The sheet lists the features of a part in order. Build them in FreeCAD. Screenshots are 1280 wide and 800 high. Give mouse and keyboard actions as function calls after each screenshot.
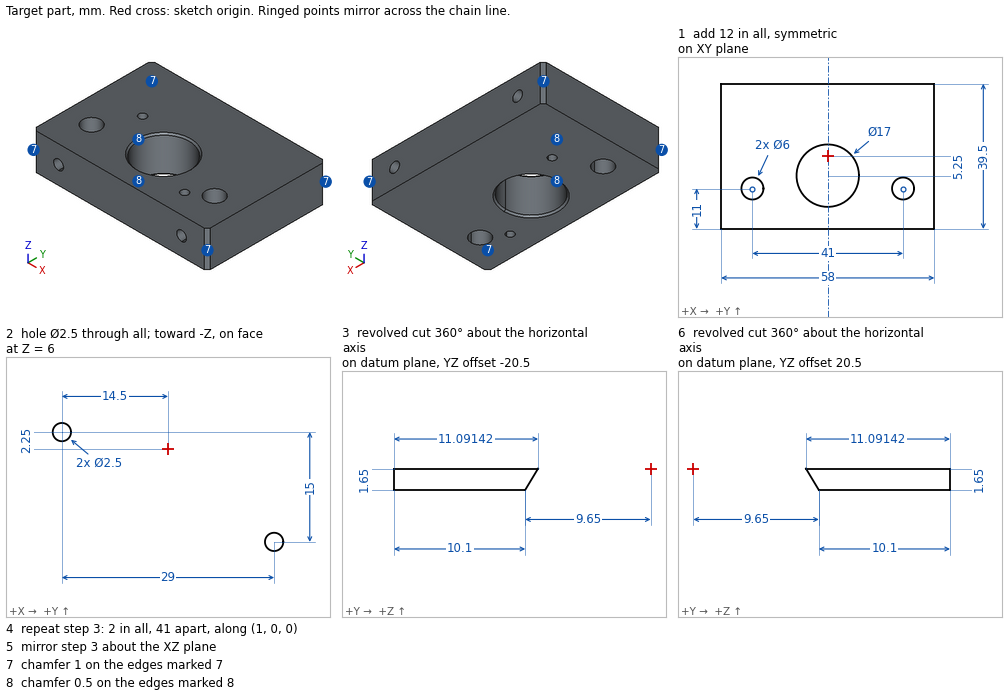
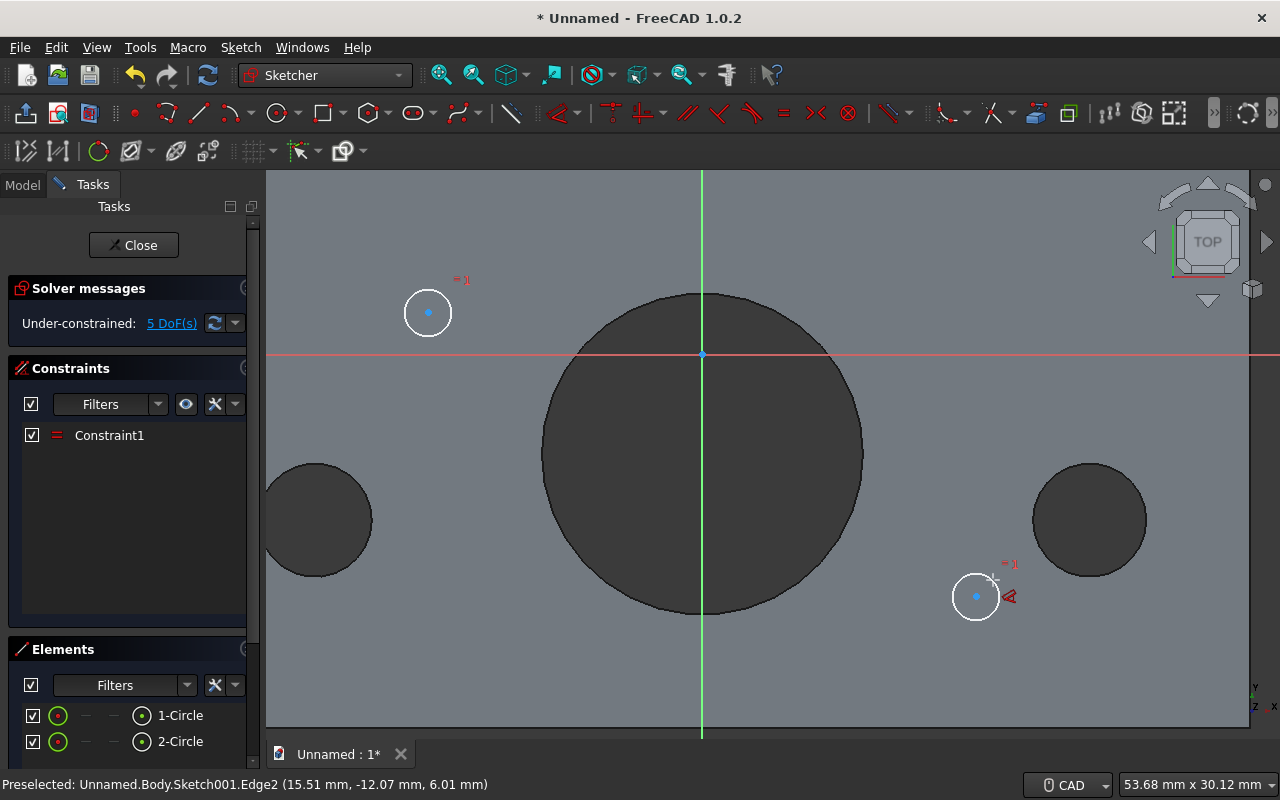
click(444, 296)
click(466, 273)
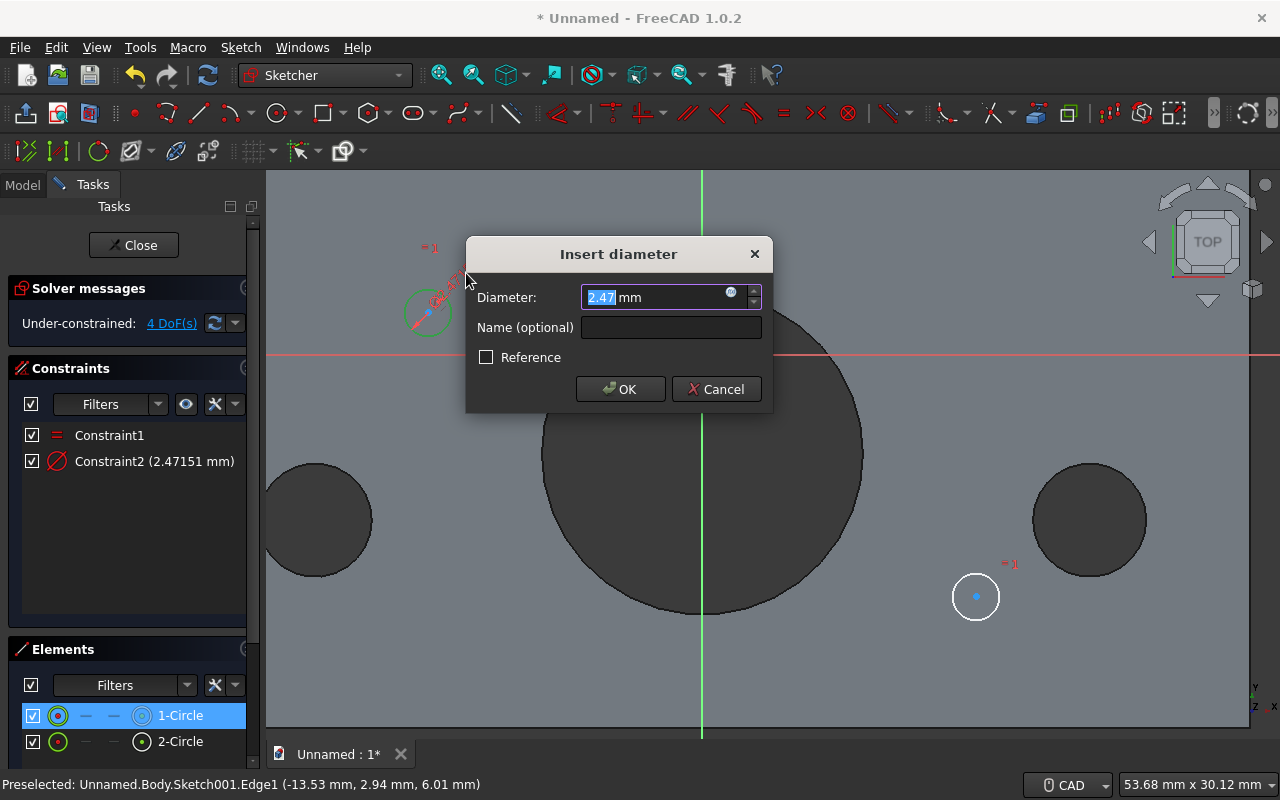
text(2.5)
key(Return)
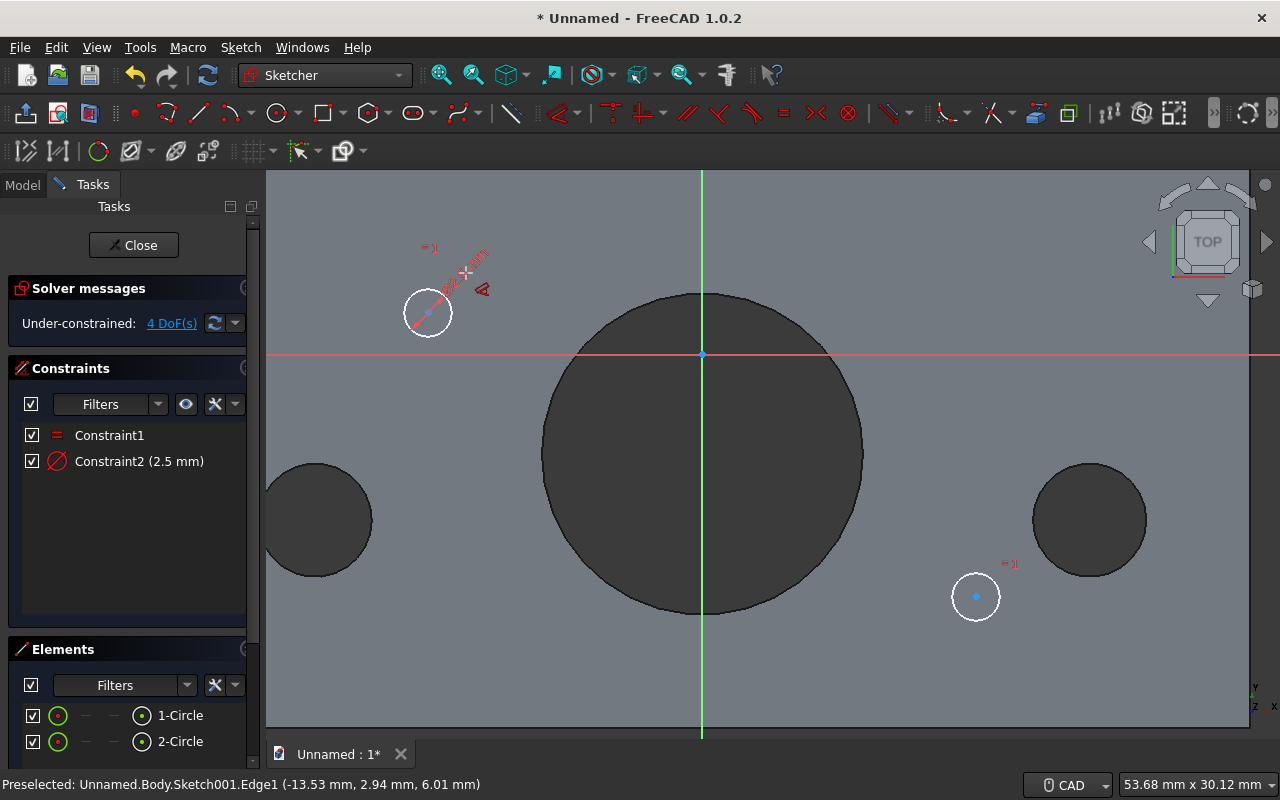
click(428, 313)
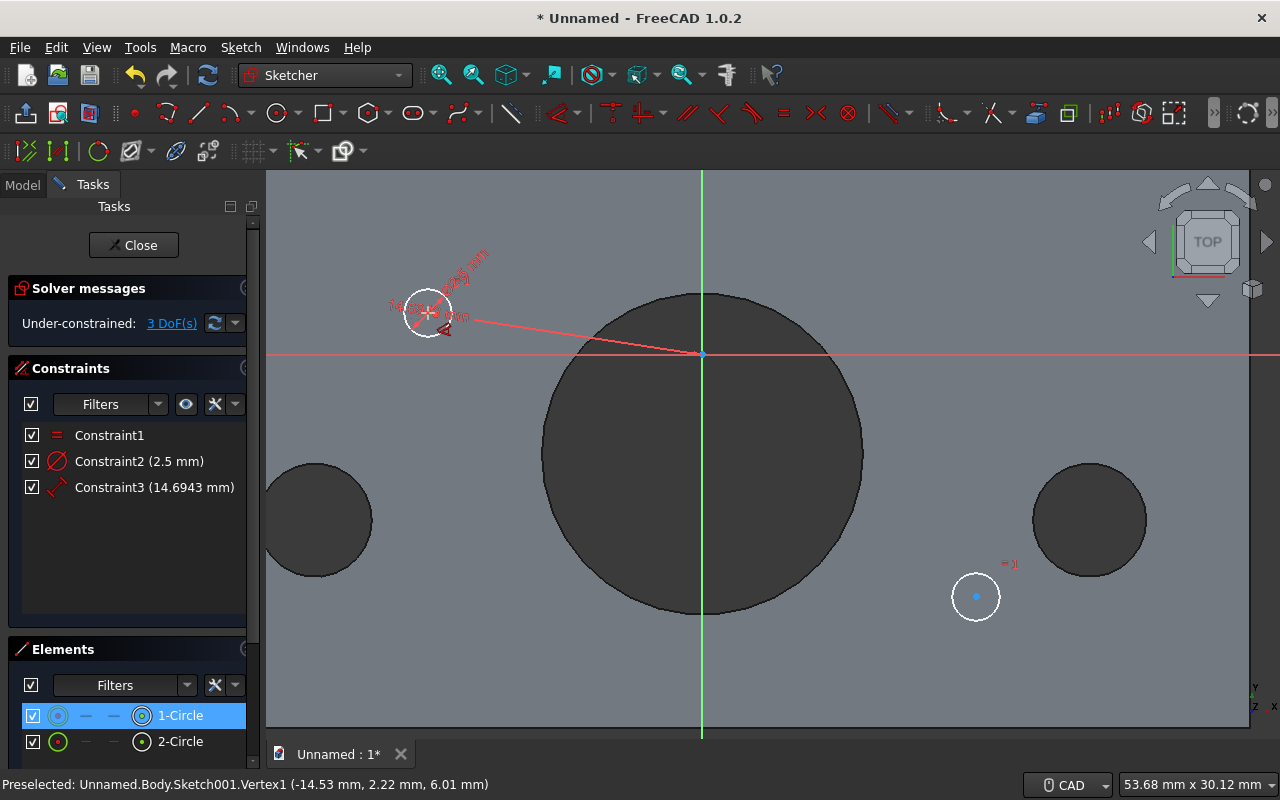
click(976, 597)
click(576, 631)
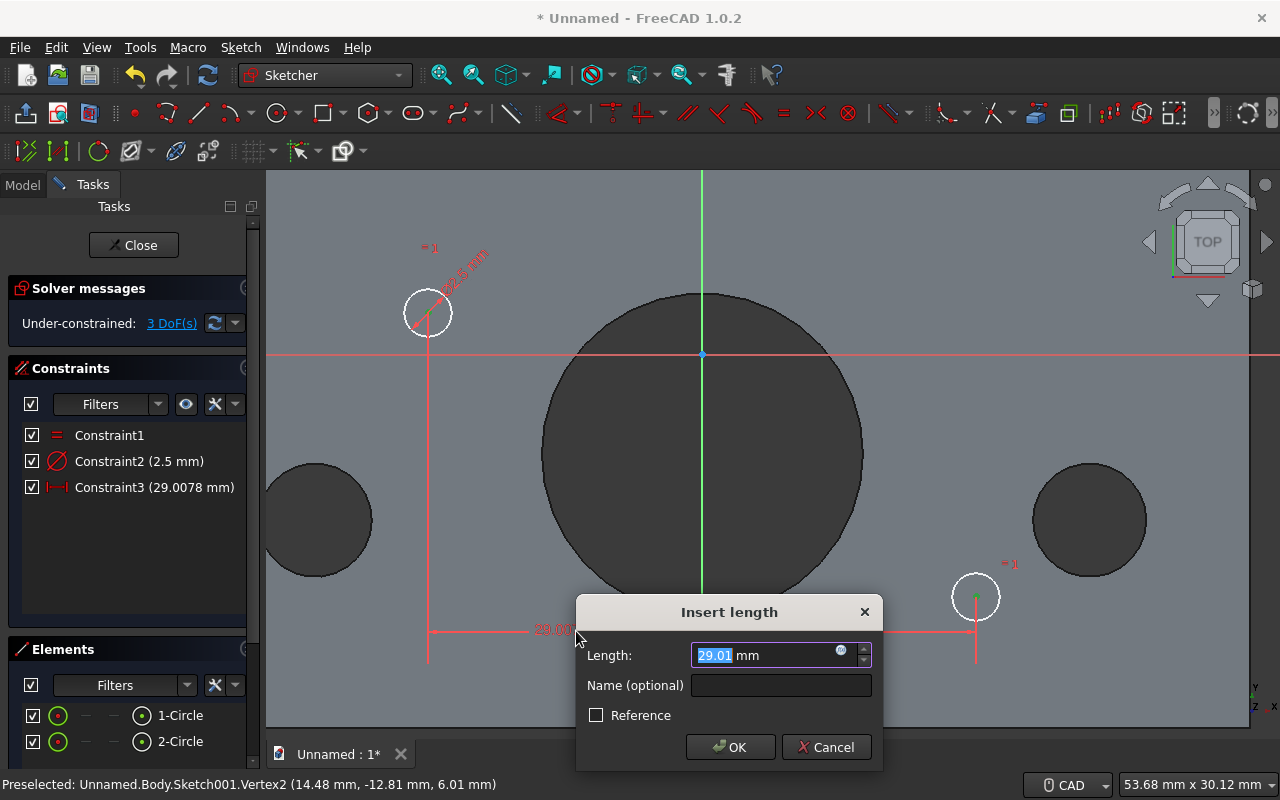
text(29)
key(Return)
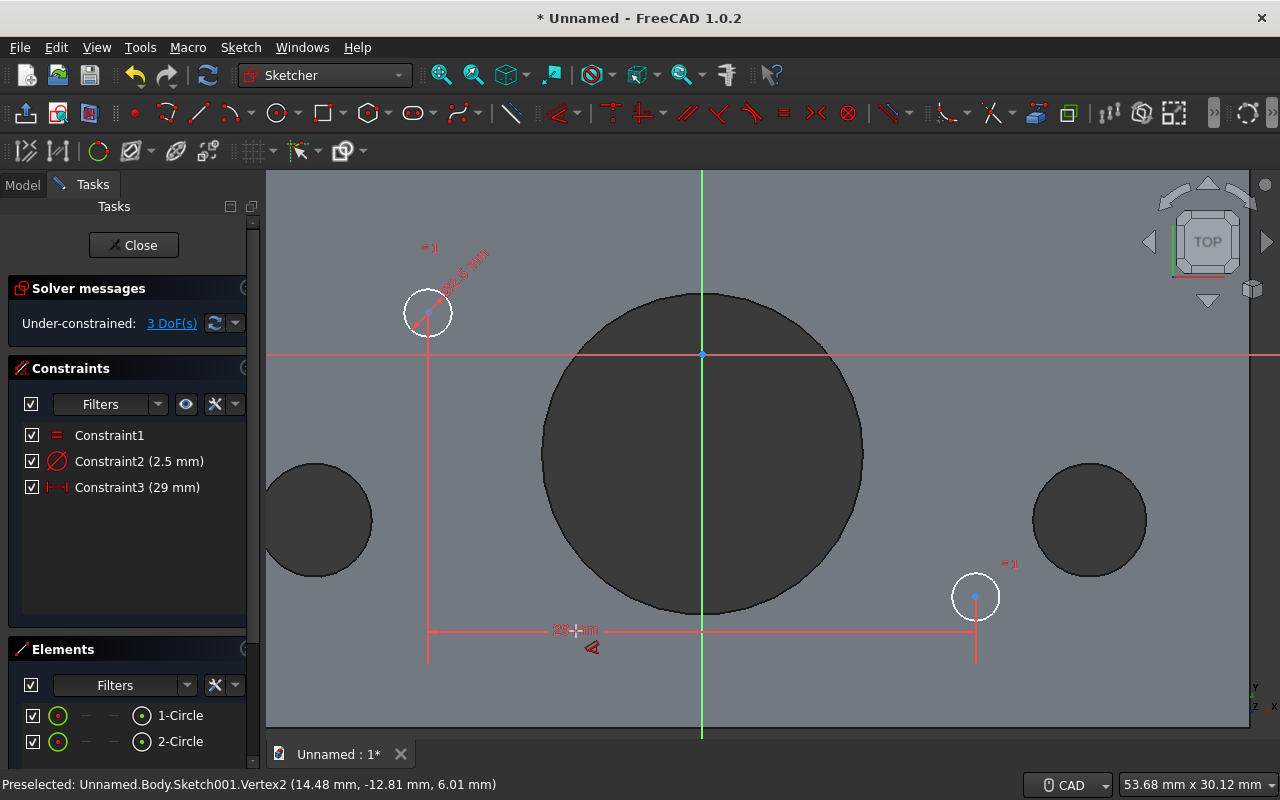
click(428, 313)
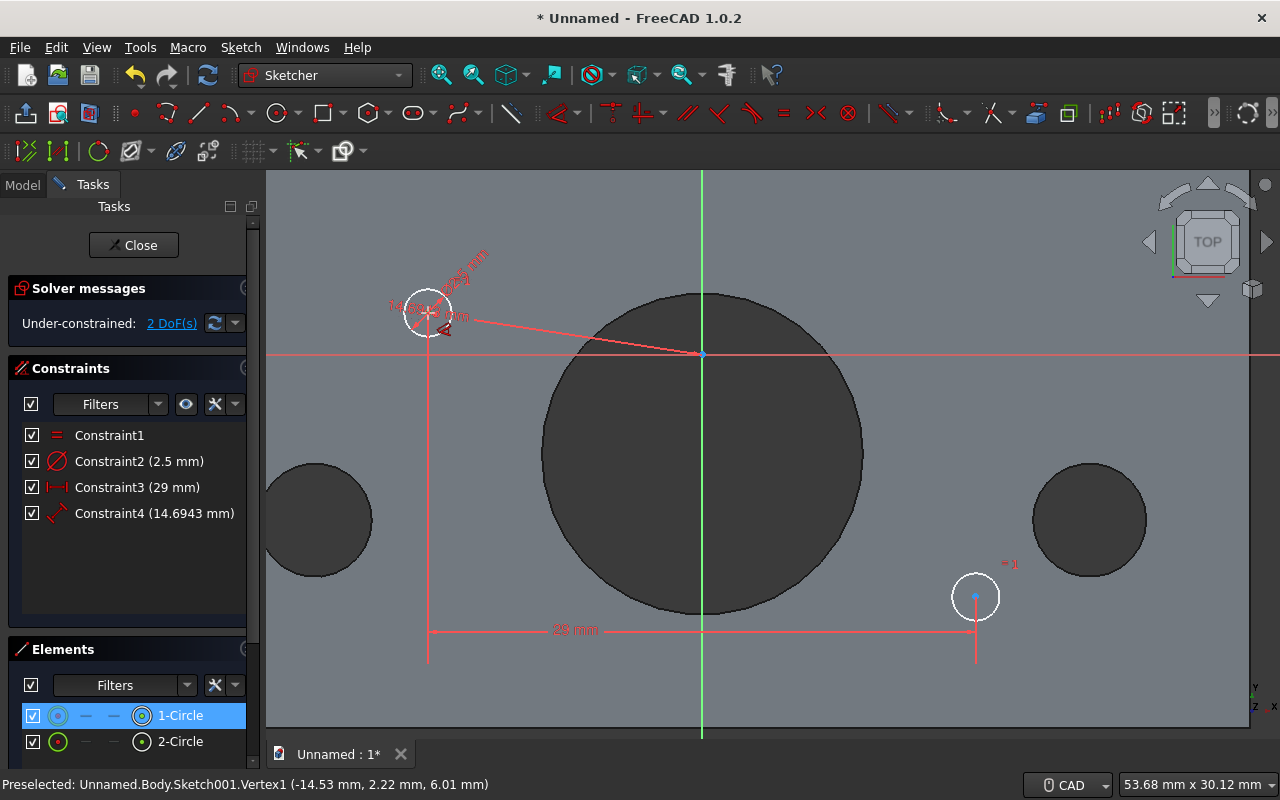
click(976, 597)
click(394, 455)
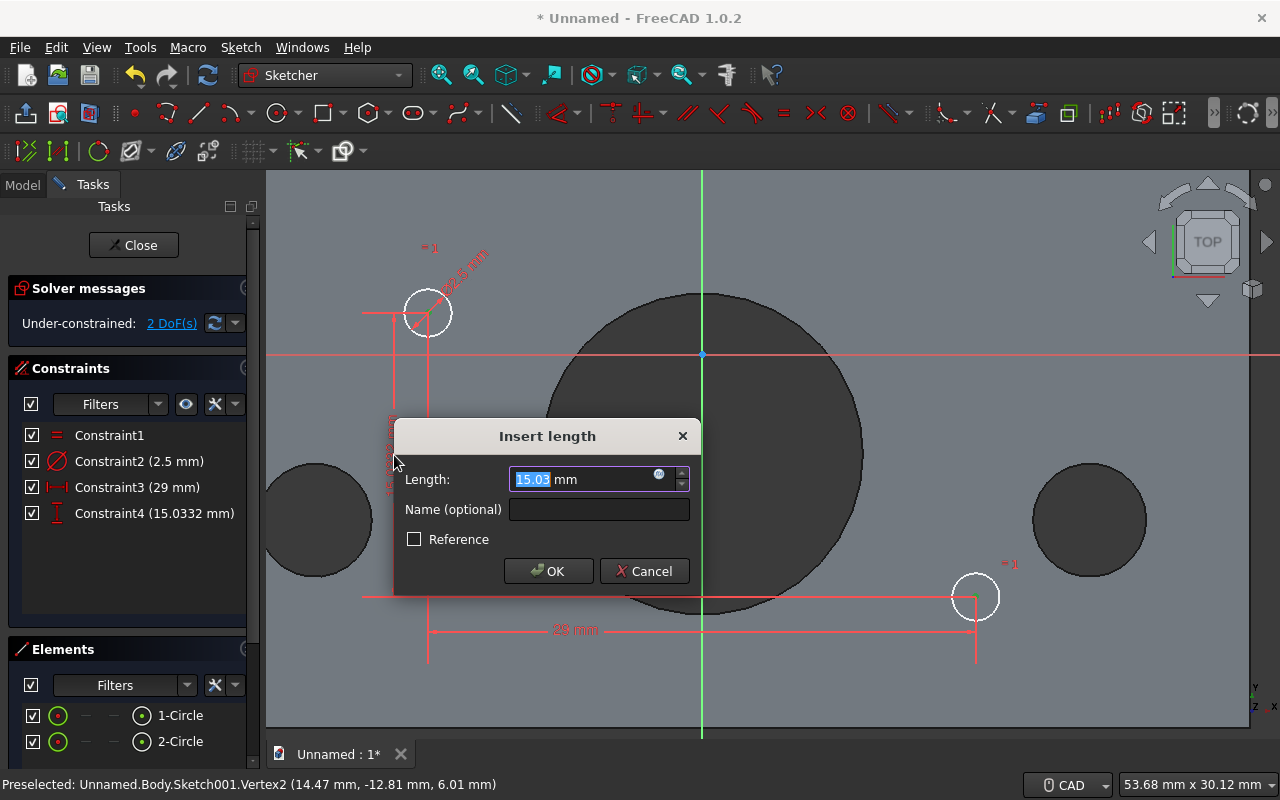
text(15)
key(Return)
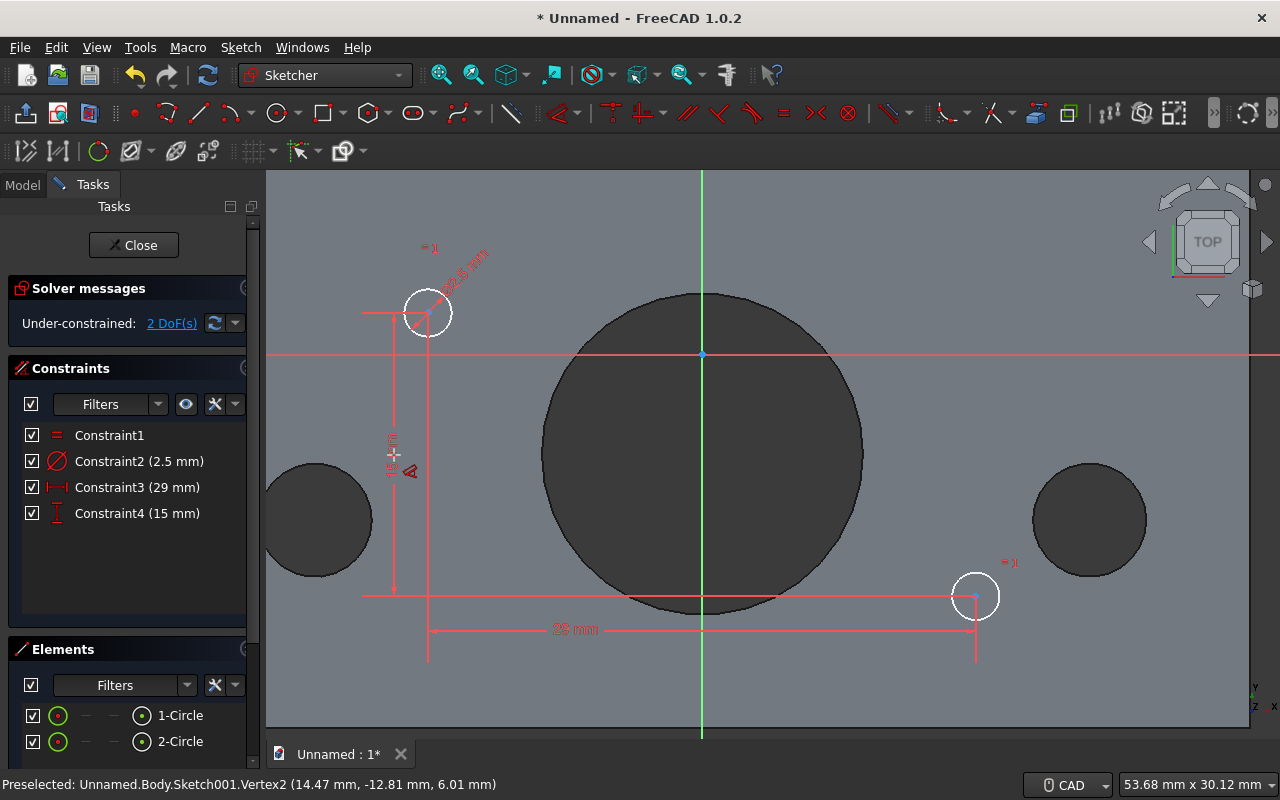
click(428, 313)
click(565, 279)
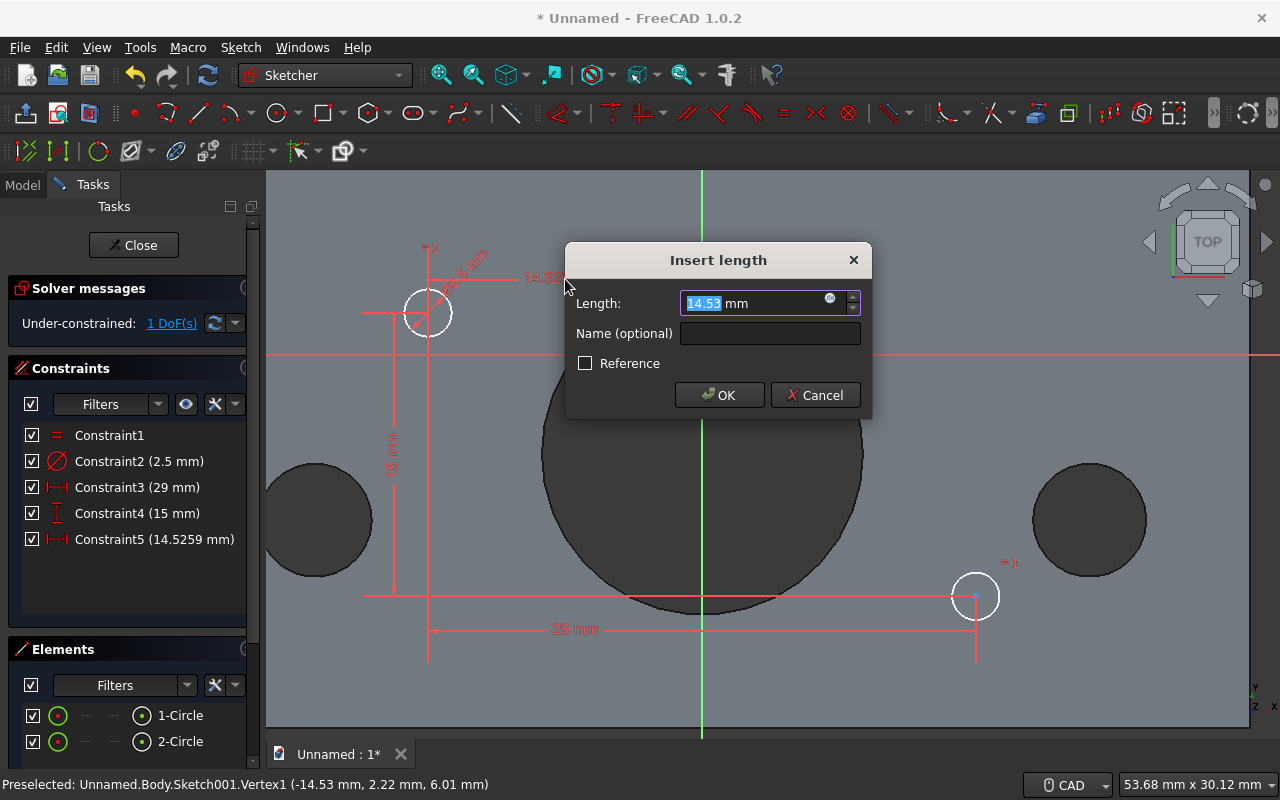
text(14.5)
key(Return)